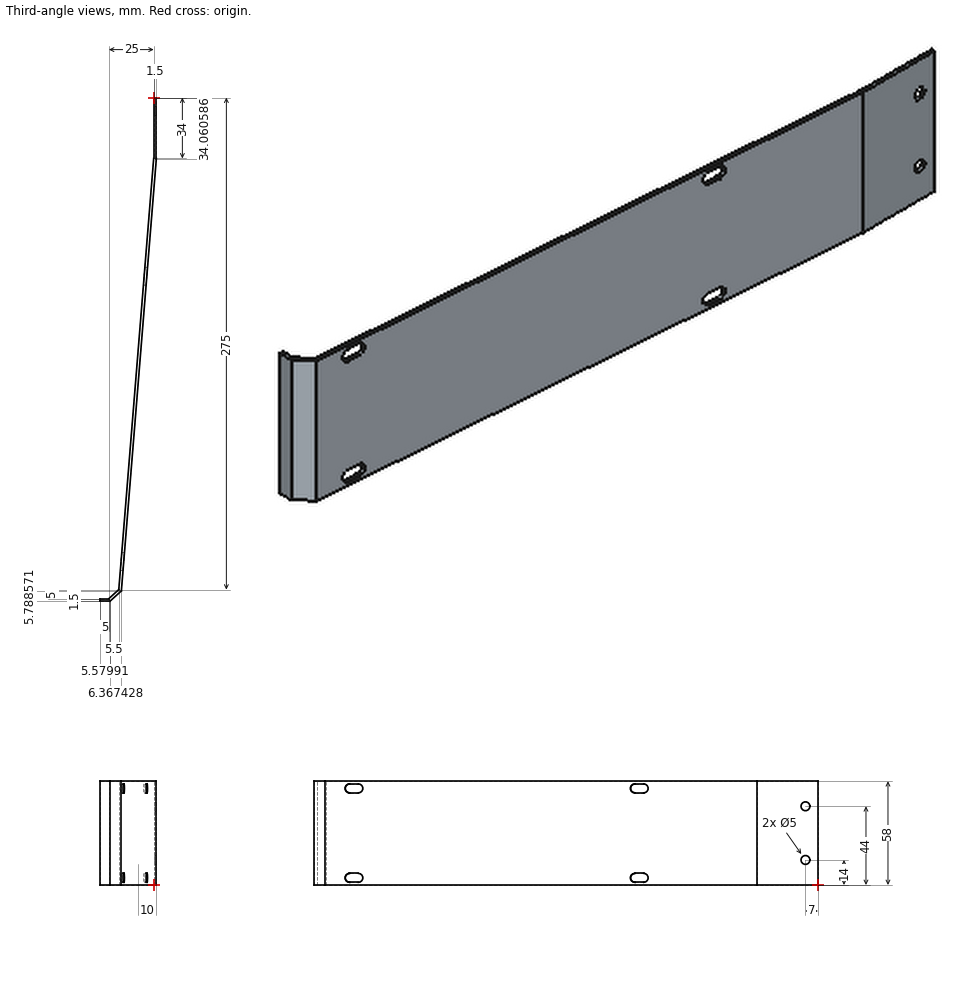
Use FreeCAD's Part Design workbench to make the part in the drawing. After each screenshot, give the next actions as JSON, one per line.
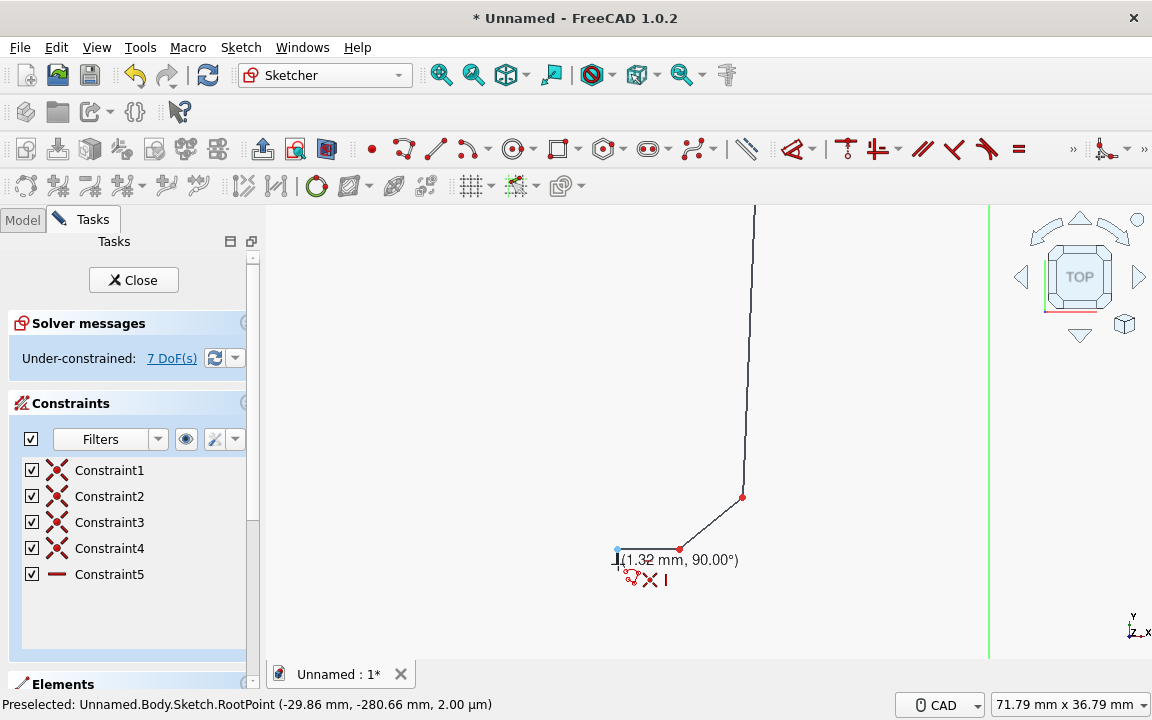
{"action": "left_click", "coordinate": [617, 563]}
{"action": "left_click", "coordinate": [688, 563]}
{"action": "left_click", "coordinate": [766, 491]}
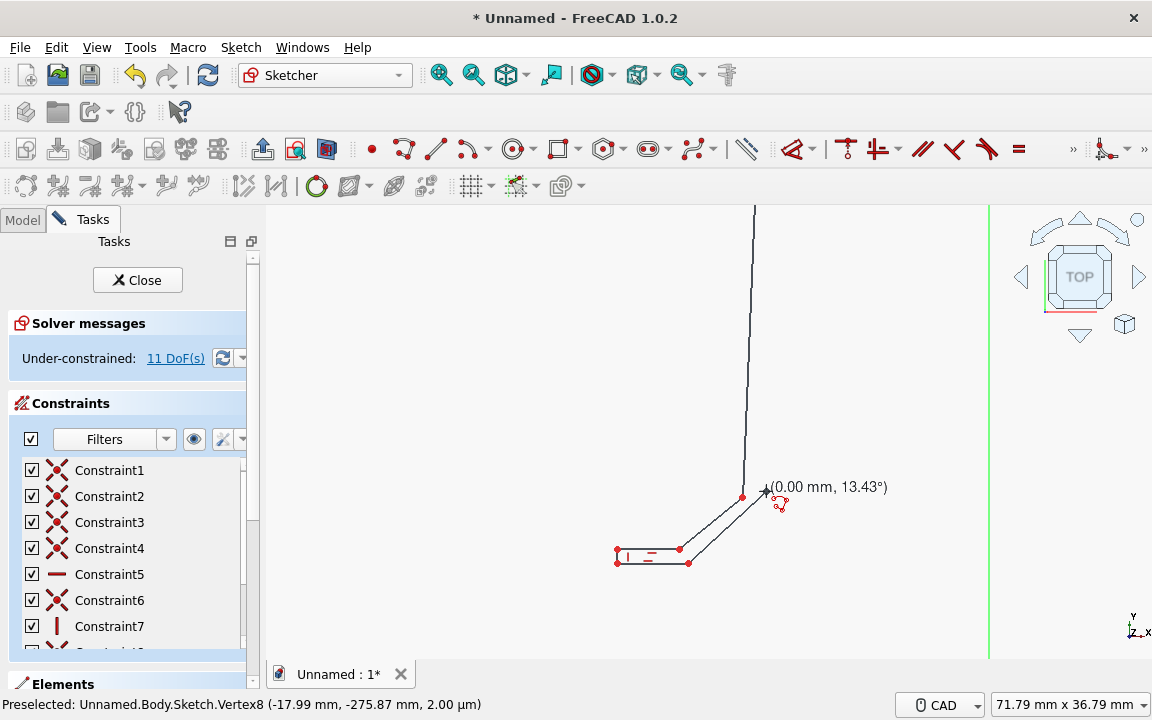
{"action": "scroll", "coordinate": [627, 561], "scroll_direction": "down", "scroll_amount": 13}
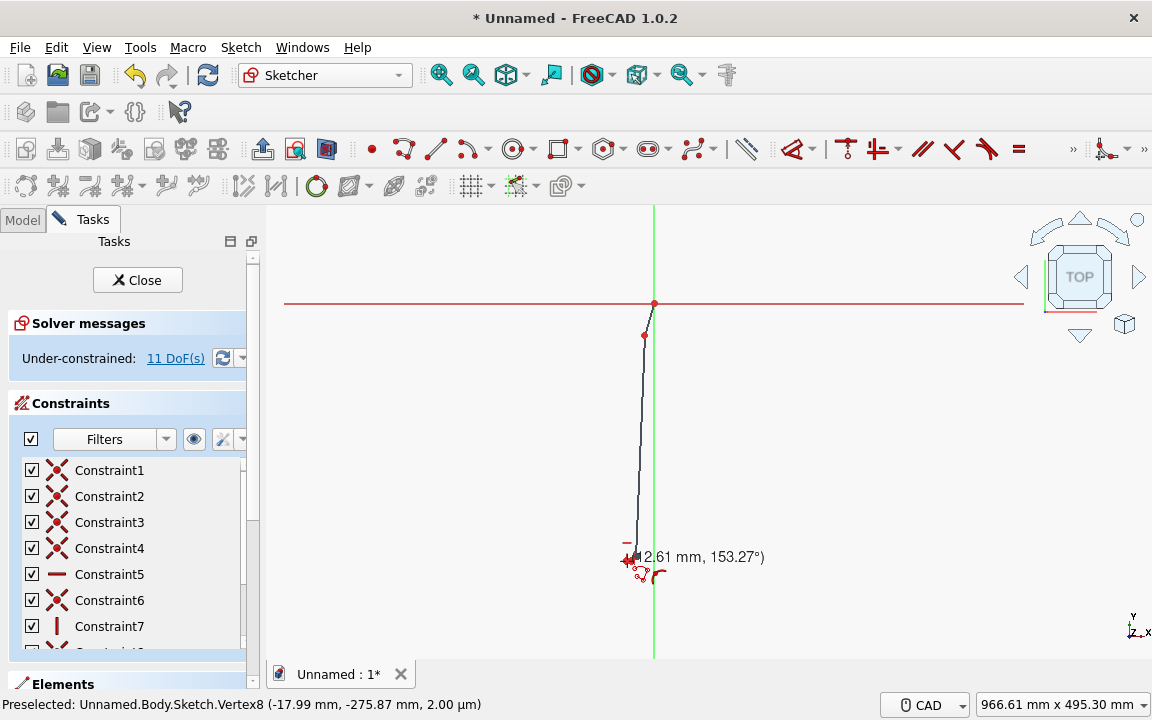
{"action": "scroll", "coordinate": [656, 335], "scroll_direction": "up", "scroll_amount": 13}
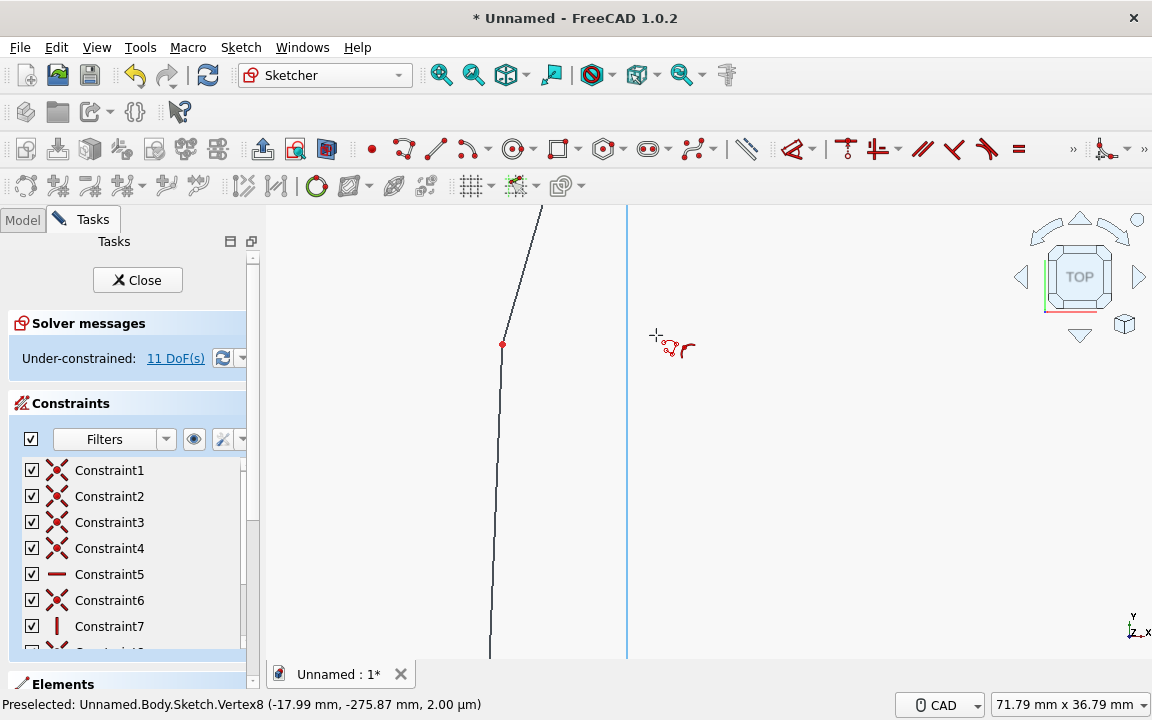
{"action": "left_click", "coordinate": [646, 332]}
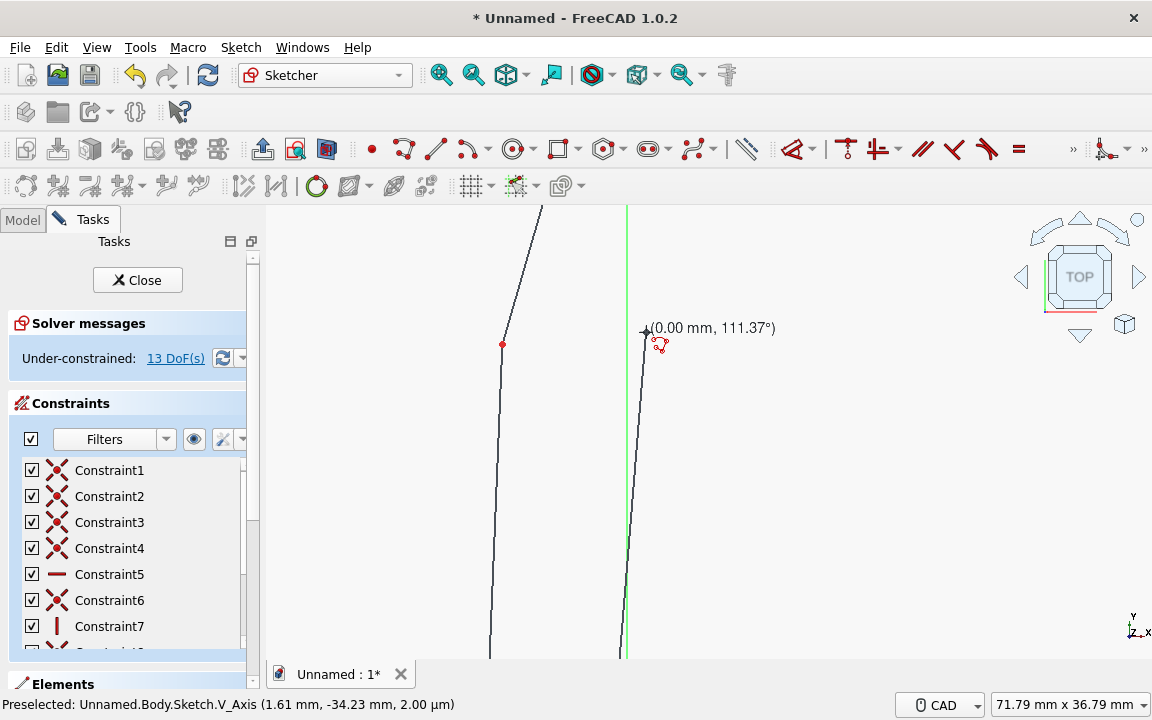
{"action": "scroll", "coordinate": [656, 334], "scroll_direction": "down", "scroll_amount": 13}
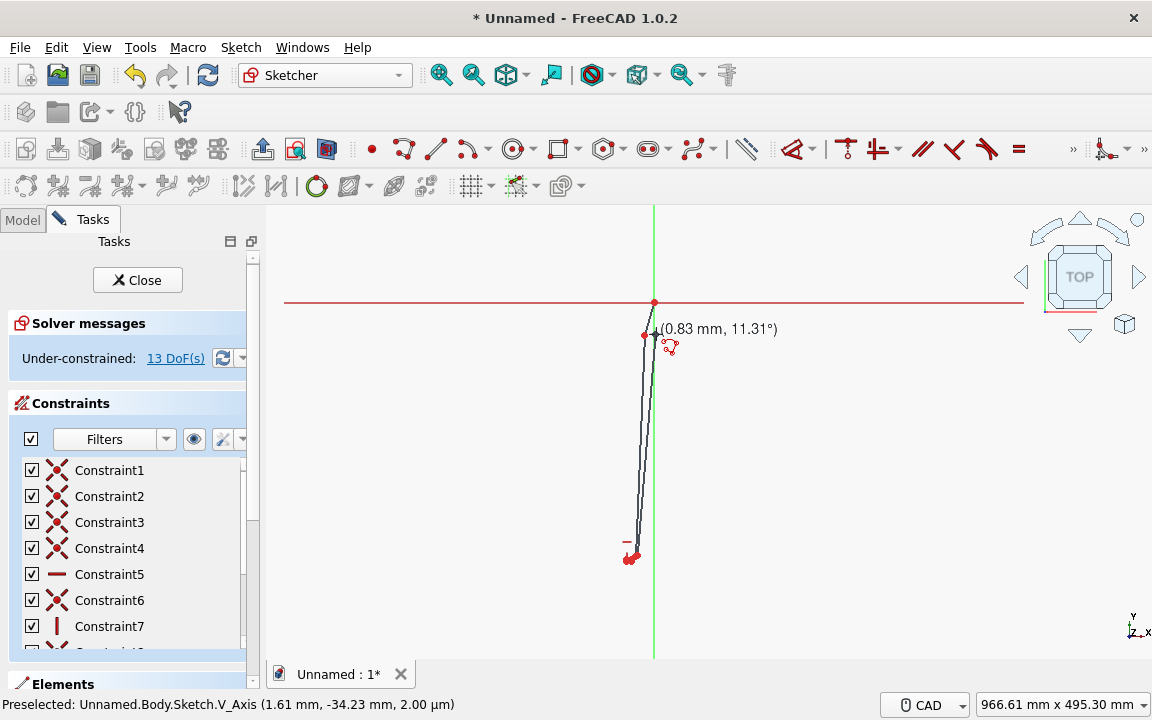
{"action": "scroll", "coordinate": [656, 303], "scroll_direction": "up", "scroll_amount": 13}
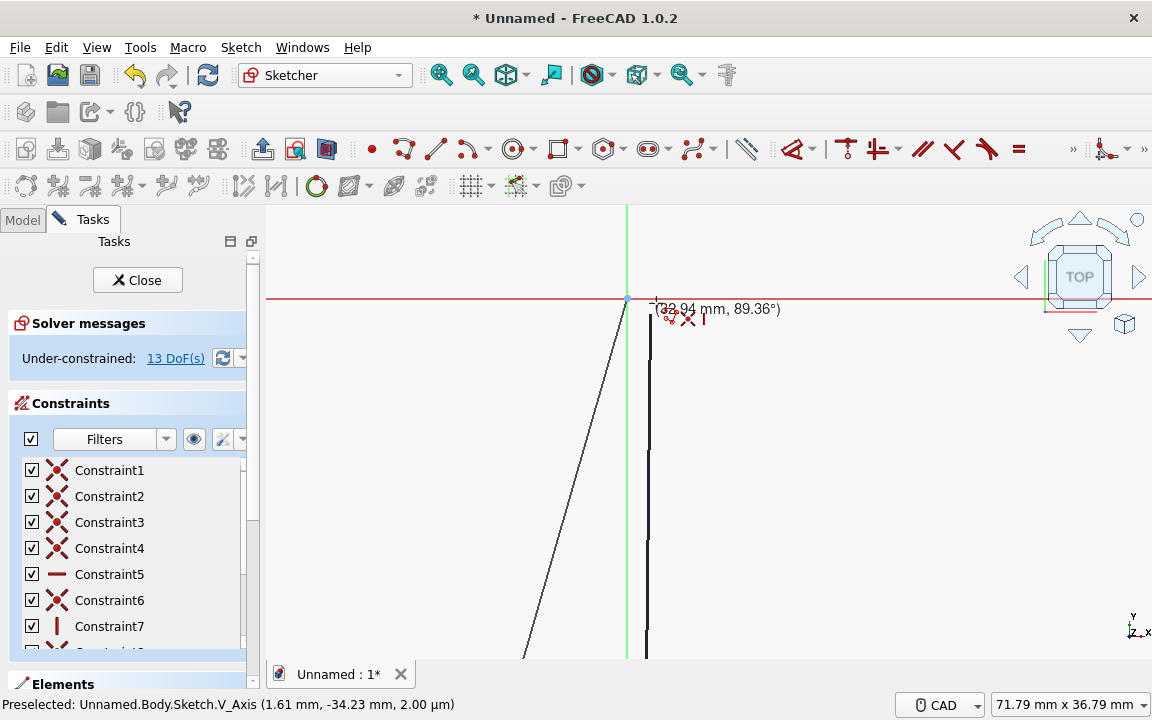
{"action": "left_click", "coordinate": [646, 308]}
{"action": "left_click", "coordinate": [627, 299]}
{"action": "key", "text": "Escape"}
{"action": "key", "text": "Escape"}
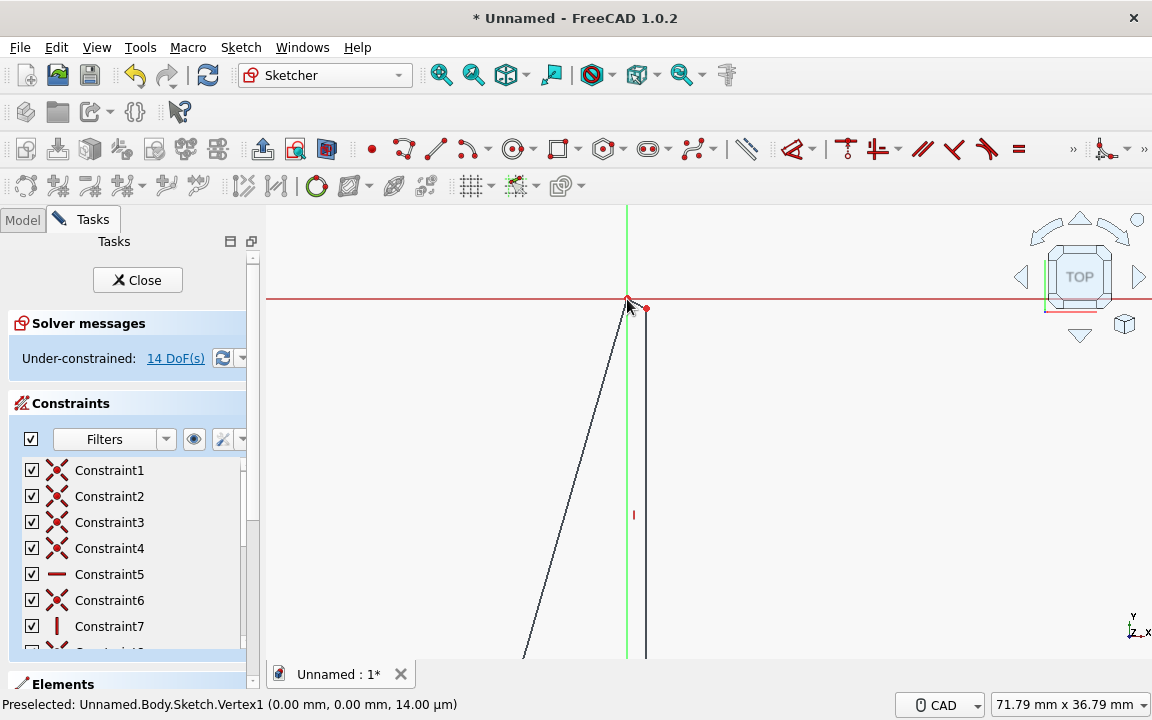
{"action": "left_click", "coordinate": [590, 429]}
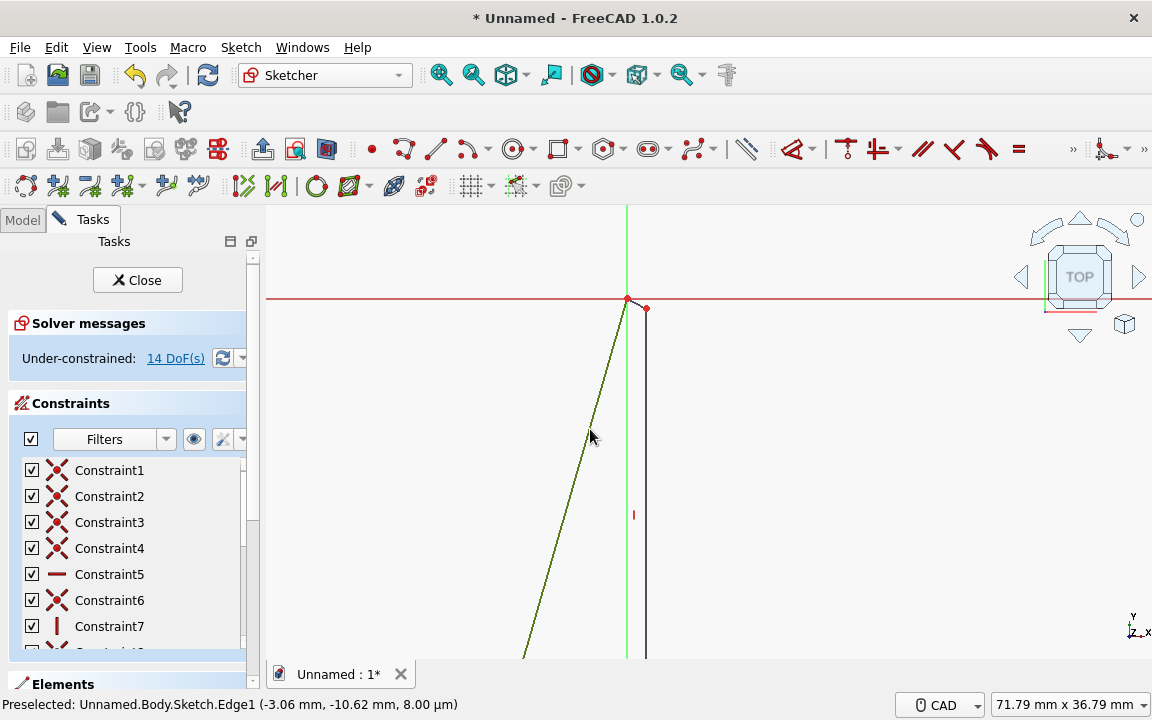
{"action": "left_click", "coordinate": [900, 150]}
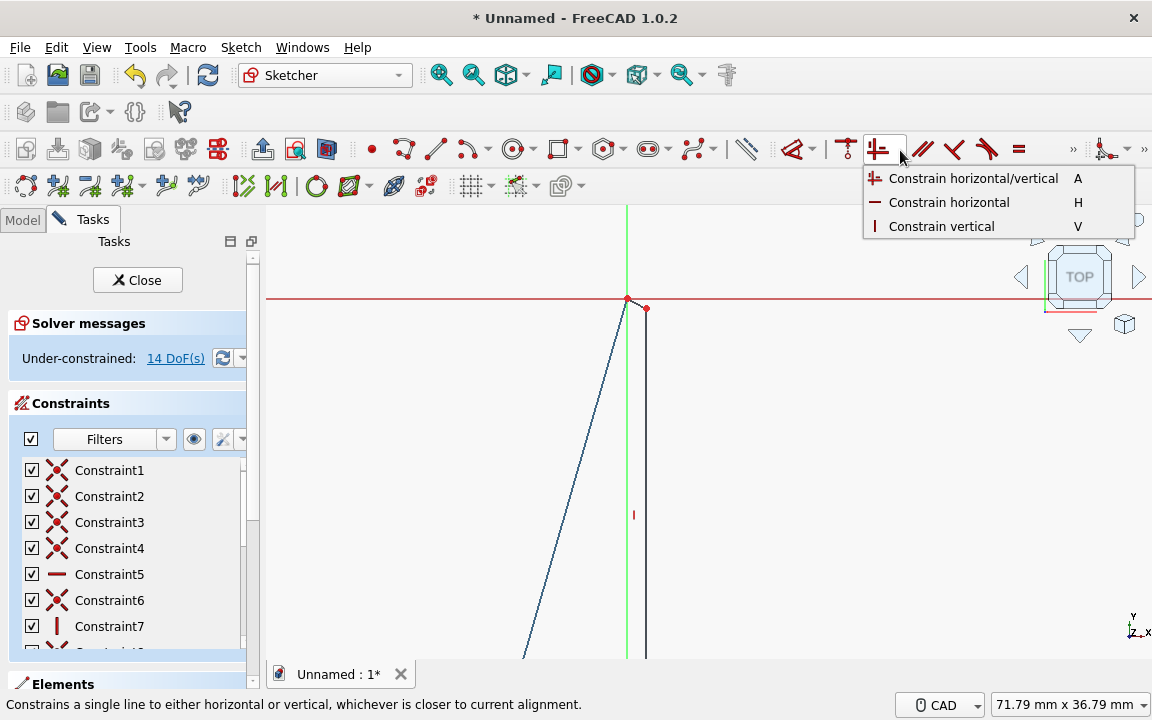
{"action": "left_click", "coordinate": [999, 226]}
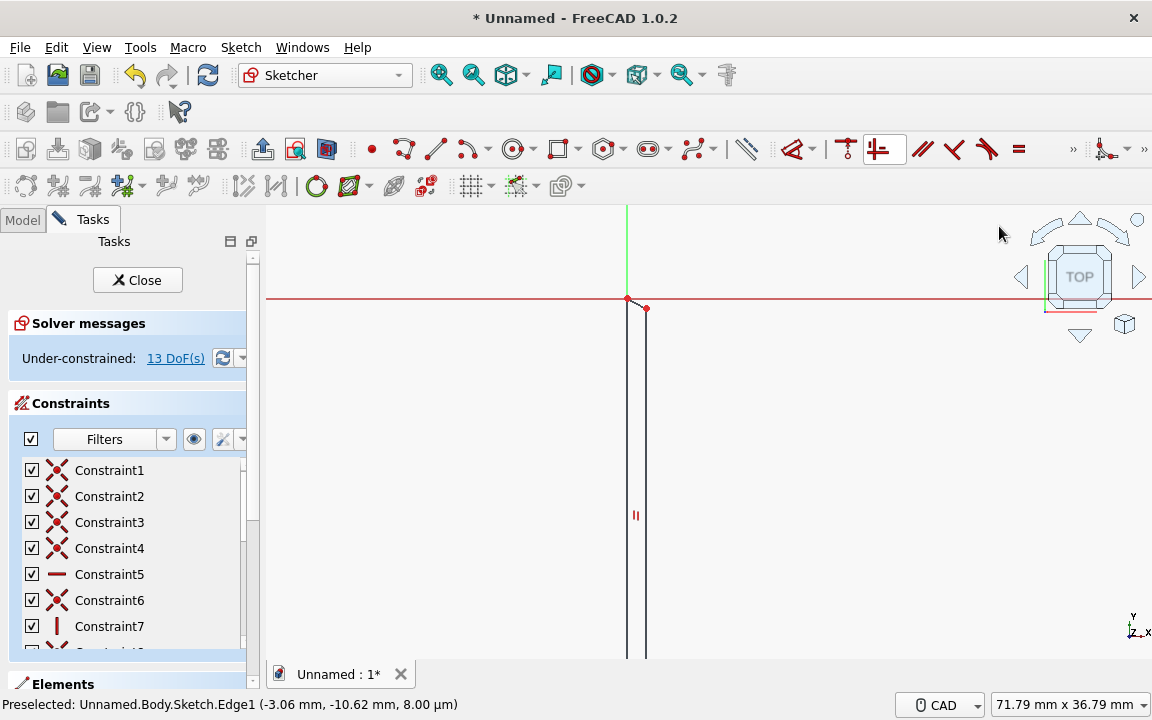
{"action": "left_click", "coordinate": [640, 306]}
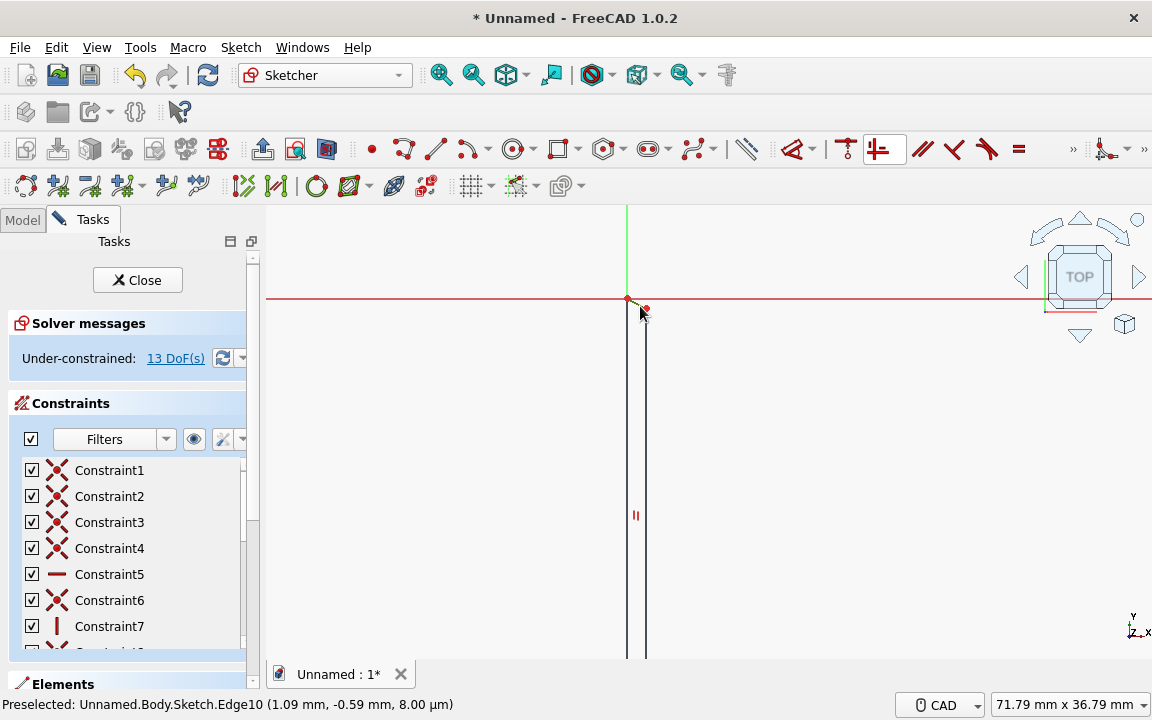
{"action": "key", "text": "h"}